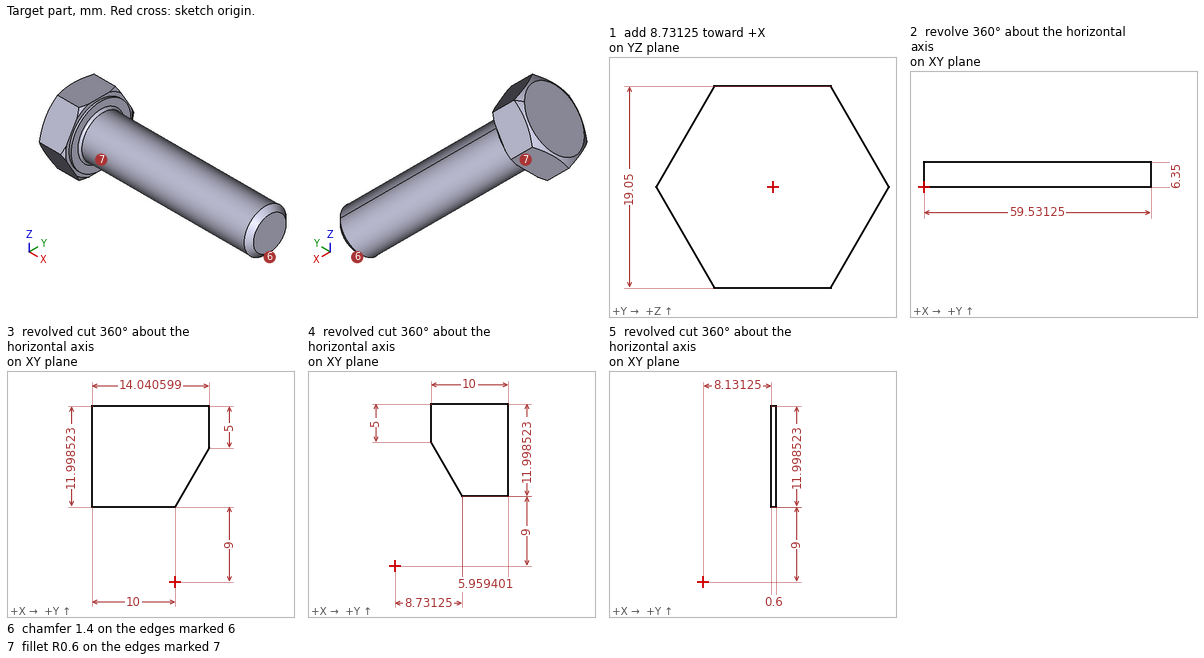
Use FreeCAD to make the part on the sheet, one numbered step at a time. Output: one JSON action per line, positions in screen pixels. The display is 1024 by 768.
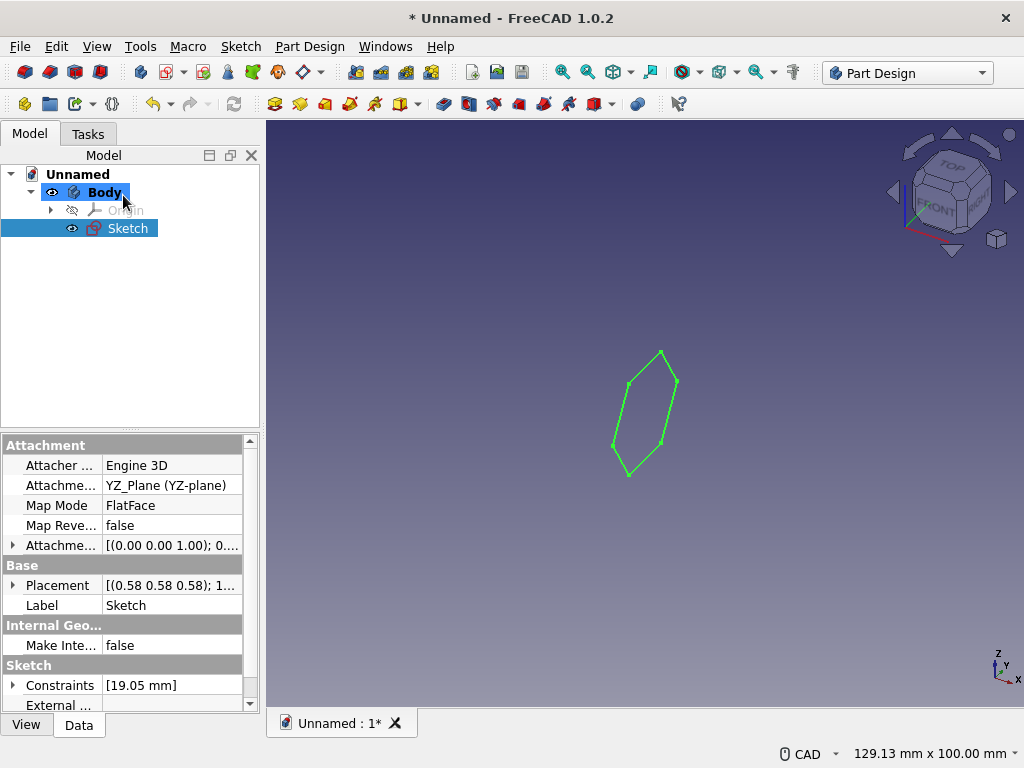
{"action": "left_click", "coordinate": [275, 104]}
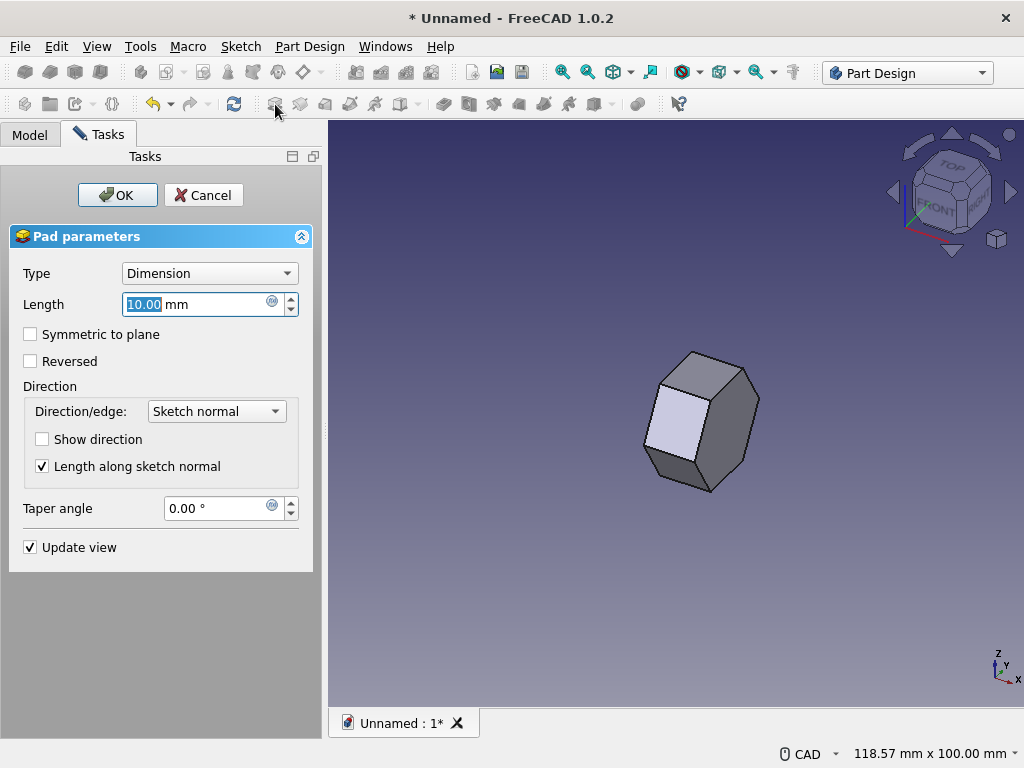
{"action": "type", "text": "8.73125"}
{"action": "key", "text": "Tab"}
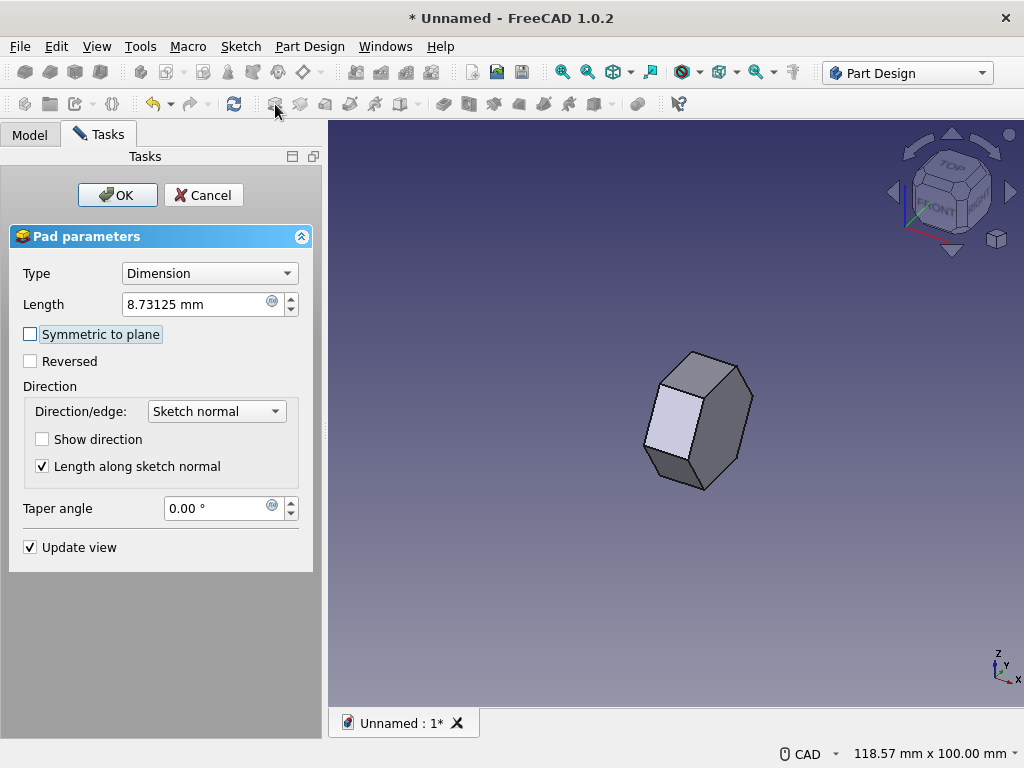
{"action": "left_click", "coordinate": [118, 195]}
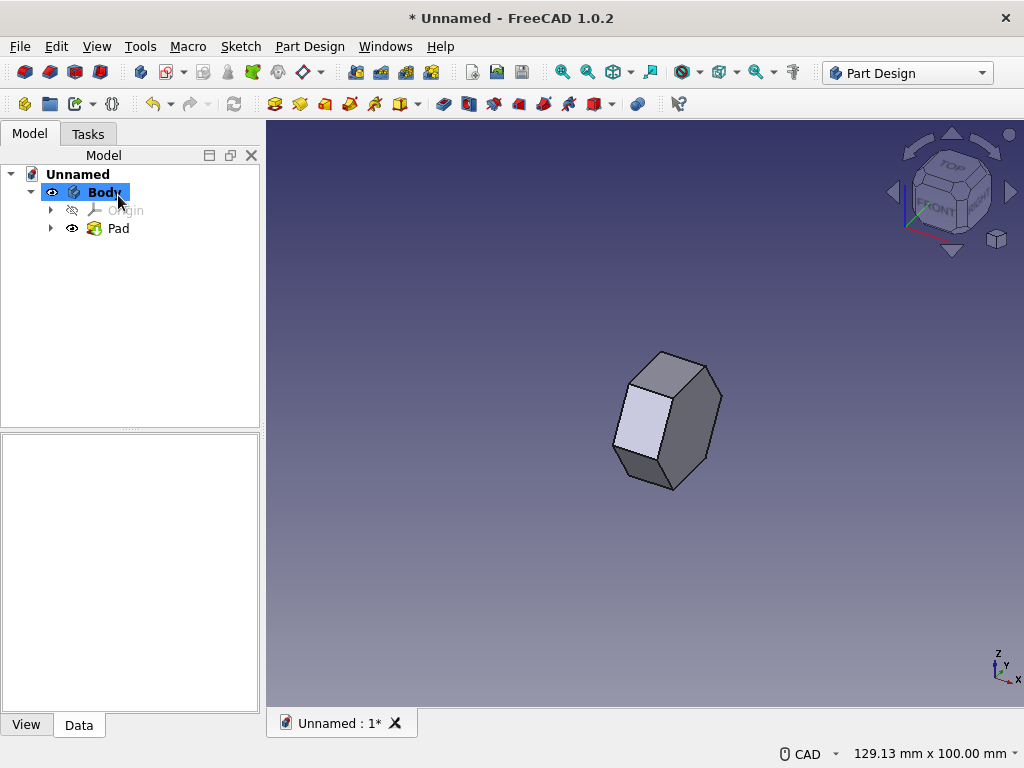
{"action": "left_click", "coordinate": [563, 72]}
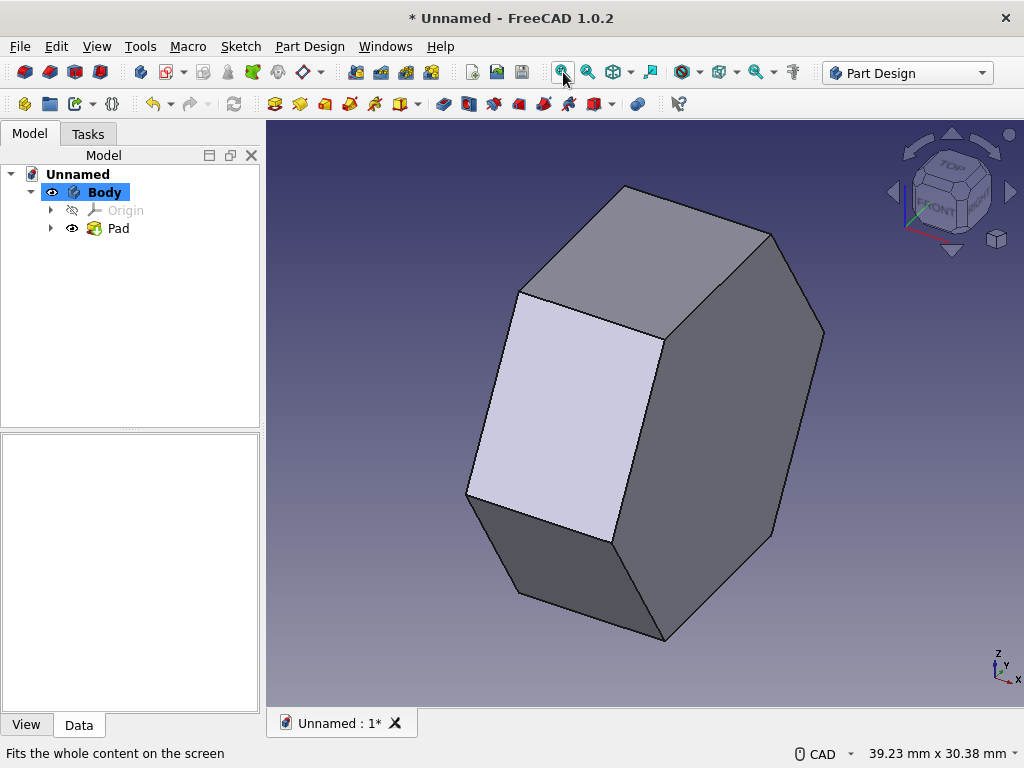
{"action": "left_click", "coordinate": [166, 72]}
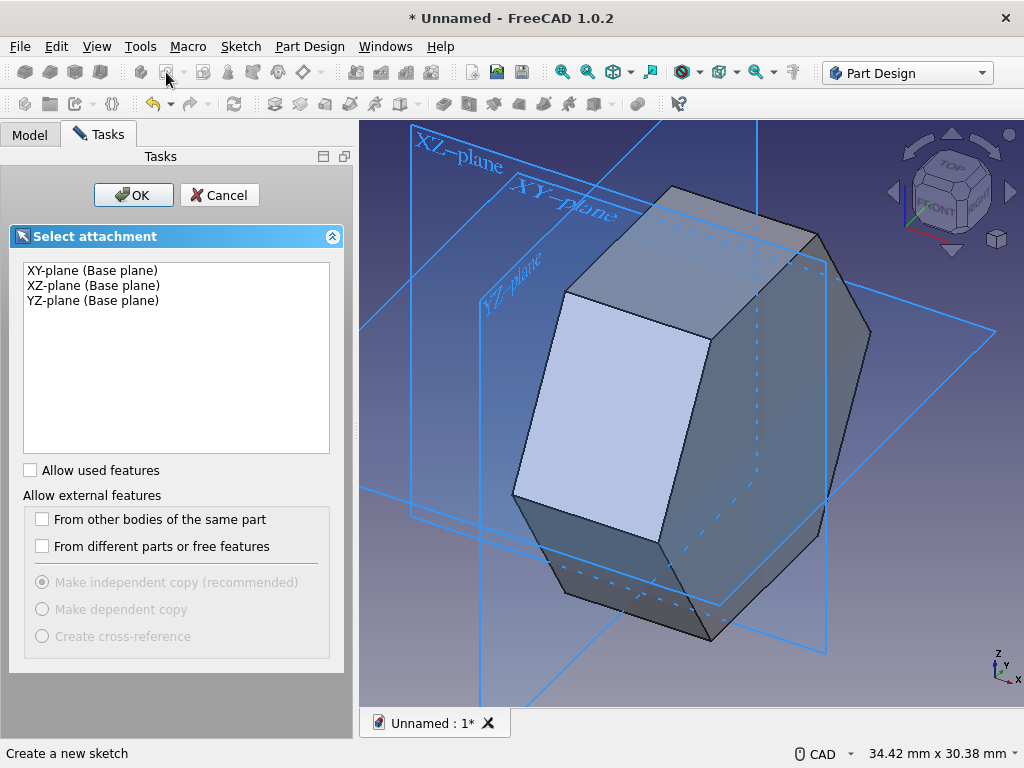
{"action": "left_click", "coordinate": [84, 270]}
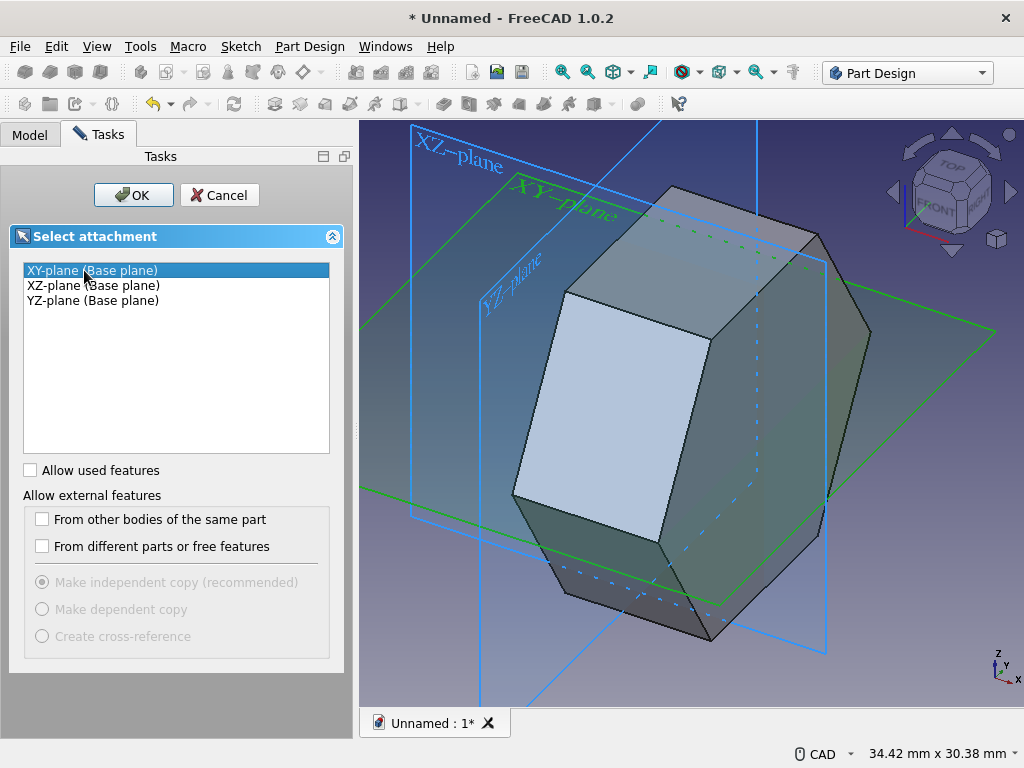
{"action": "left_click", "coordinate": [134, 195]}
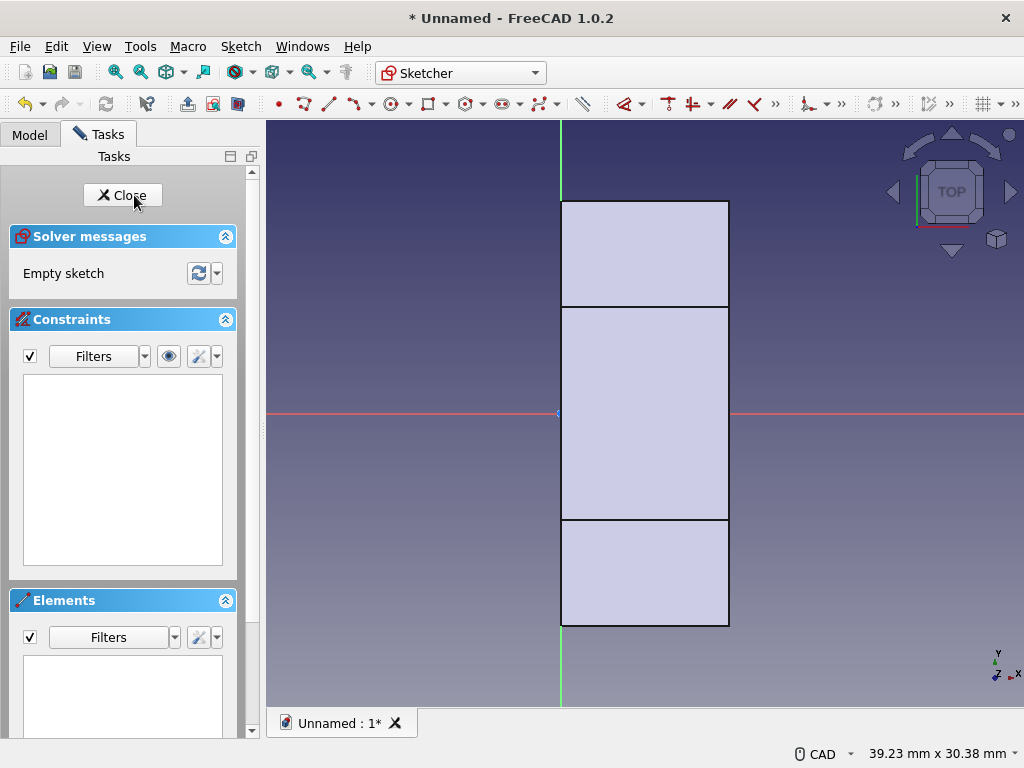
{"action": "left_click", "coordinate": [238, 104]}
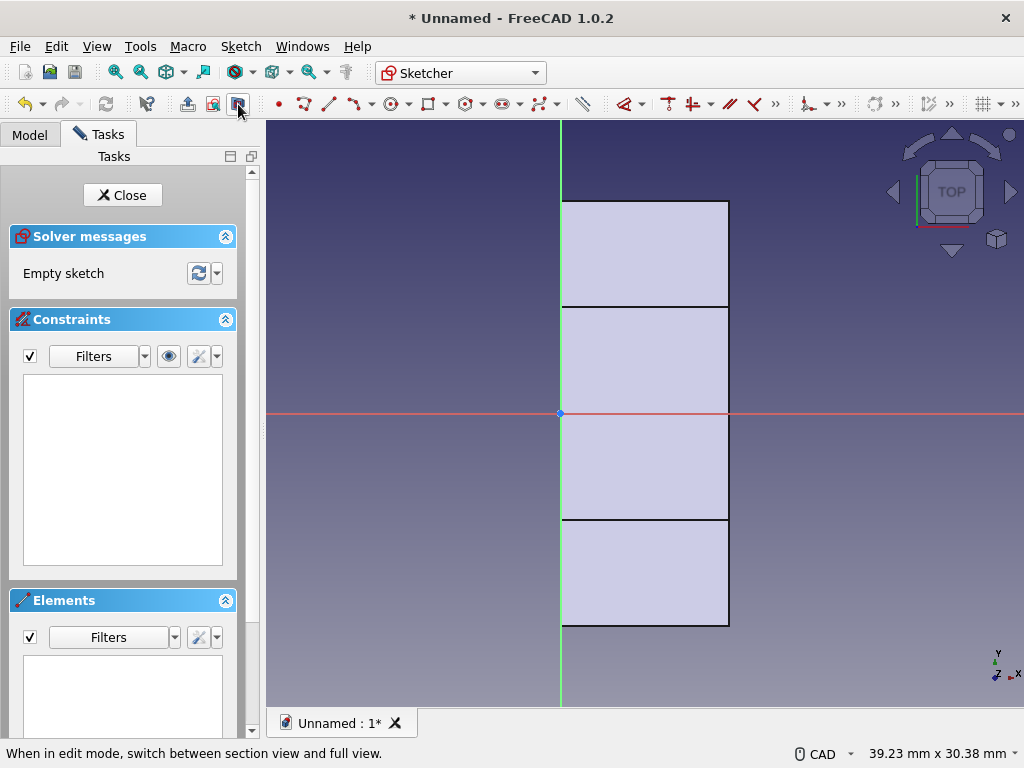
{"action": "scroll", "coordinate": [294, 449], "scroll_direction": "down", "scroll_amount": 5}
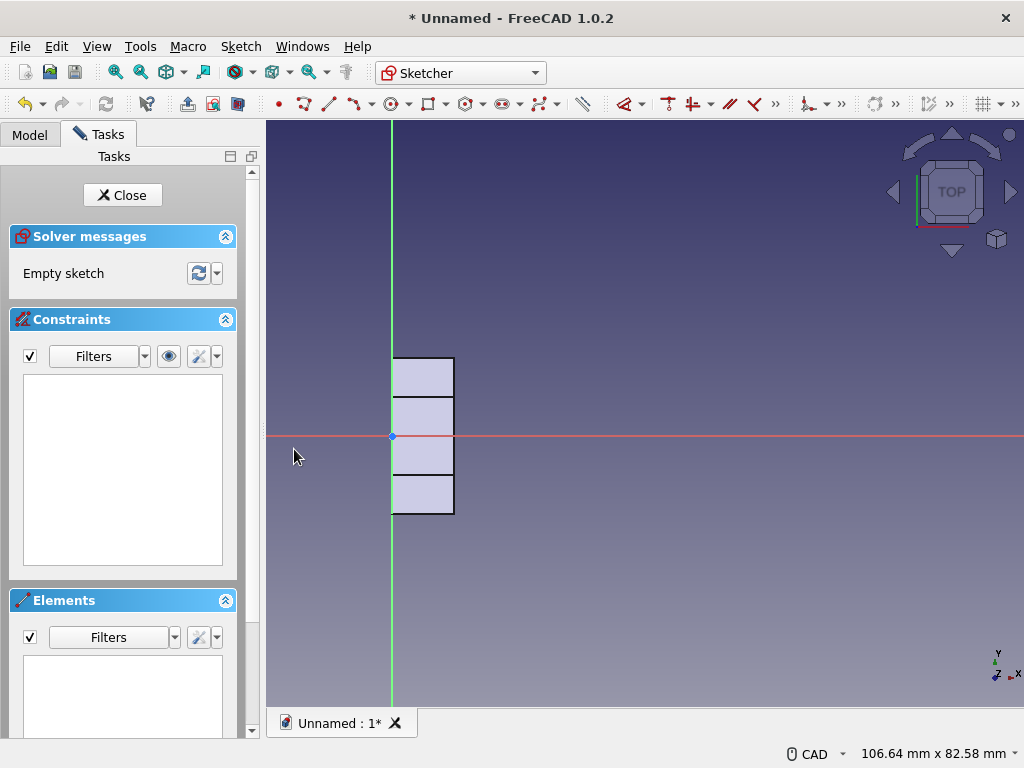
{"action": "left_click", "coordinate": [428, 104]}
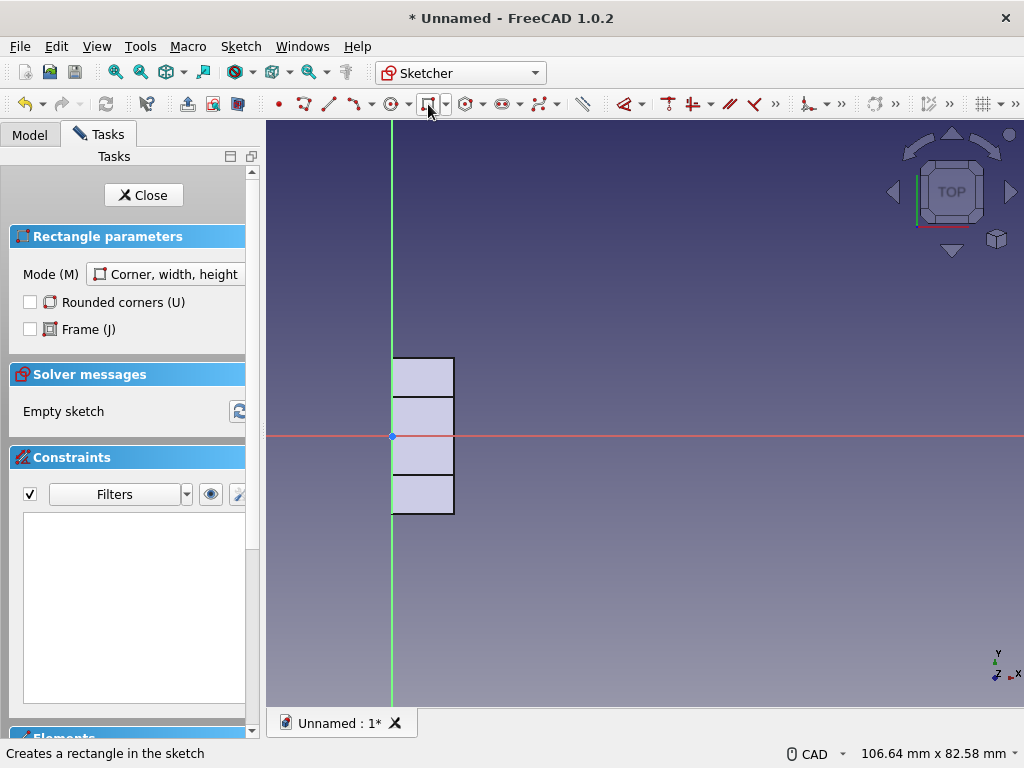
{"action": "left_click", "coordinate": [392, 436]}
{"action": "left_click", "coordinate": [815, 391]}
{"action": "key", "text": "Escape"}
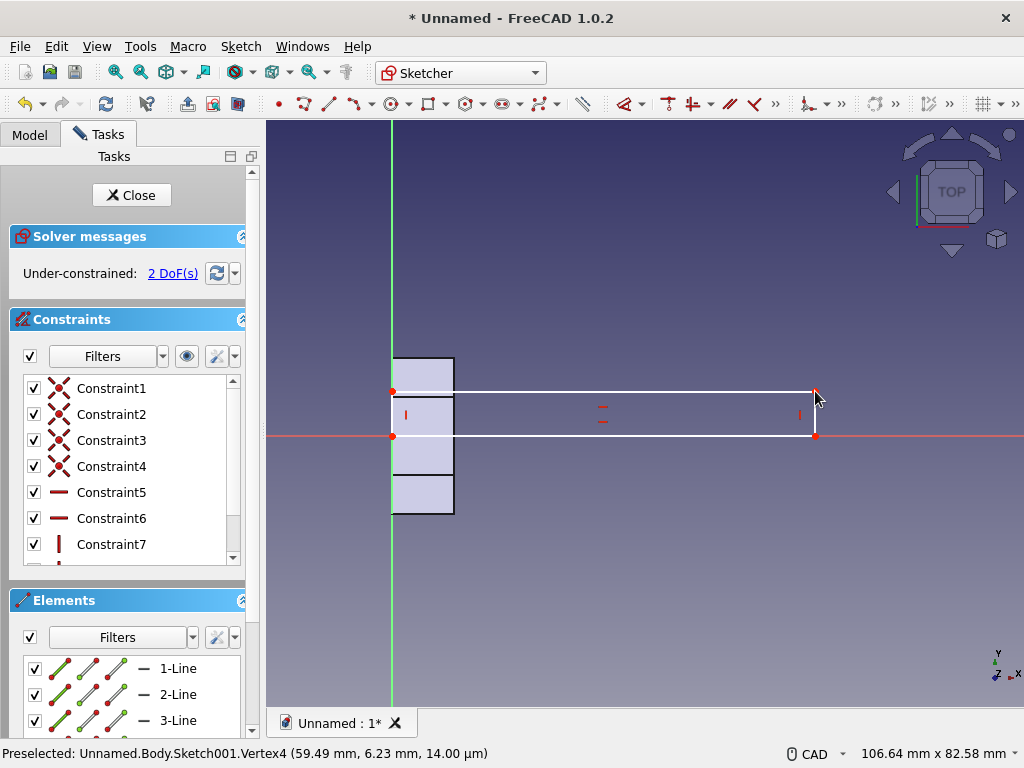
{"action": "left_click", "coordinate": [624, 104]}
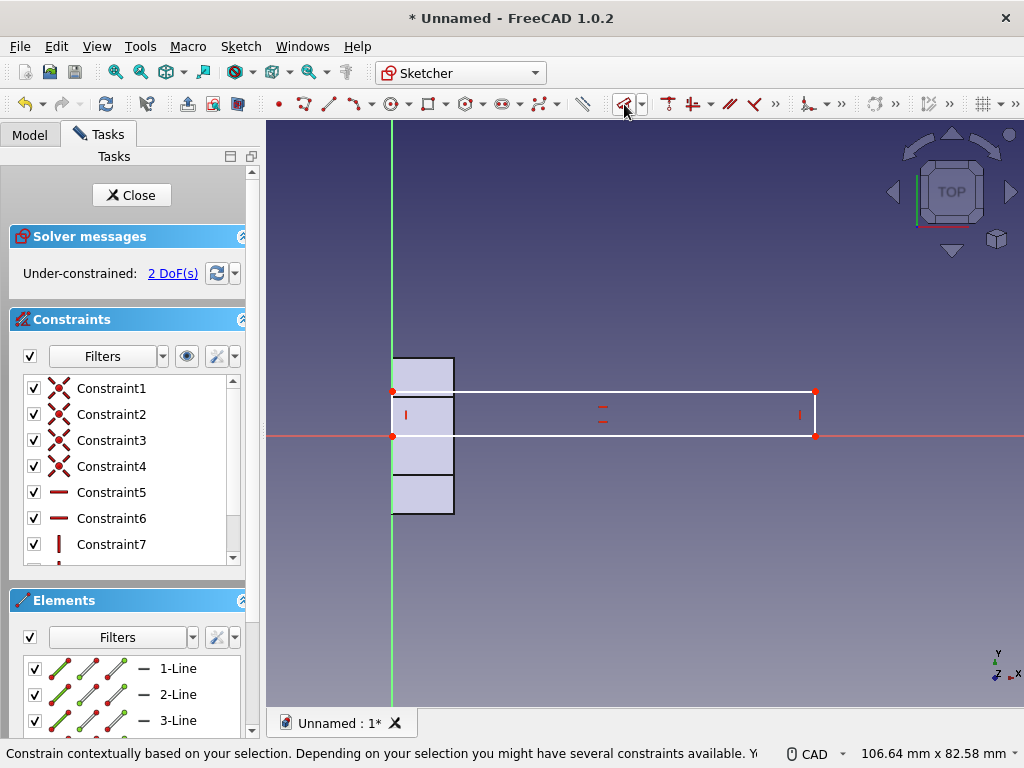
{"action": "left_click", "coordinate": [815, 423]}
{"action": "left_click", "coordinate": [849, 414]}